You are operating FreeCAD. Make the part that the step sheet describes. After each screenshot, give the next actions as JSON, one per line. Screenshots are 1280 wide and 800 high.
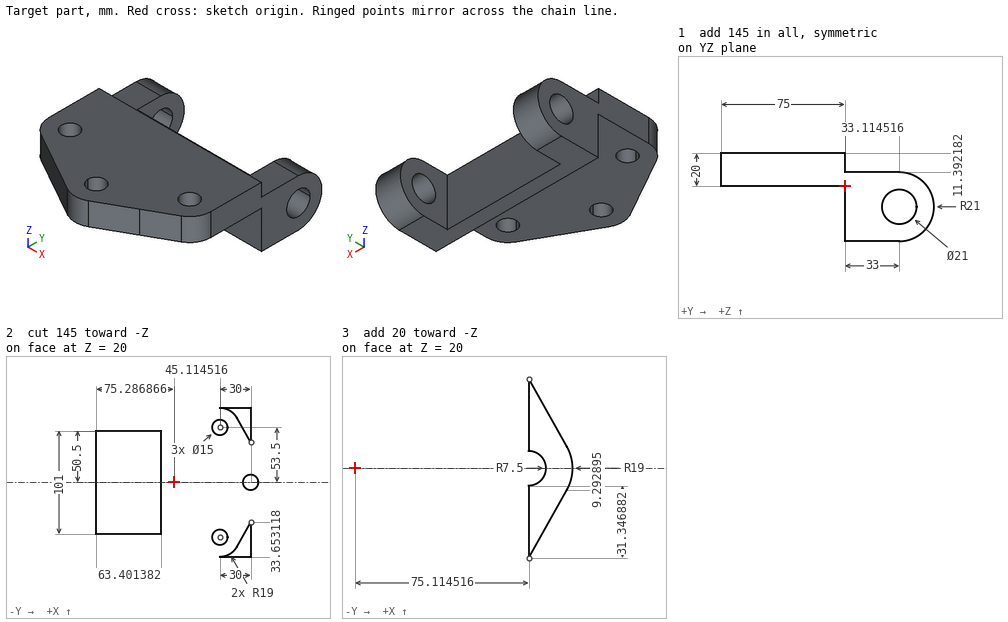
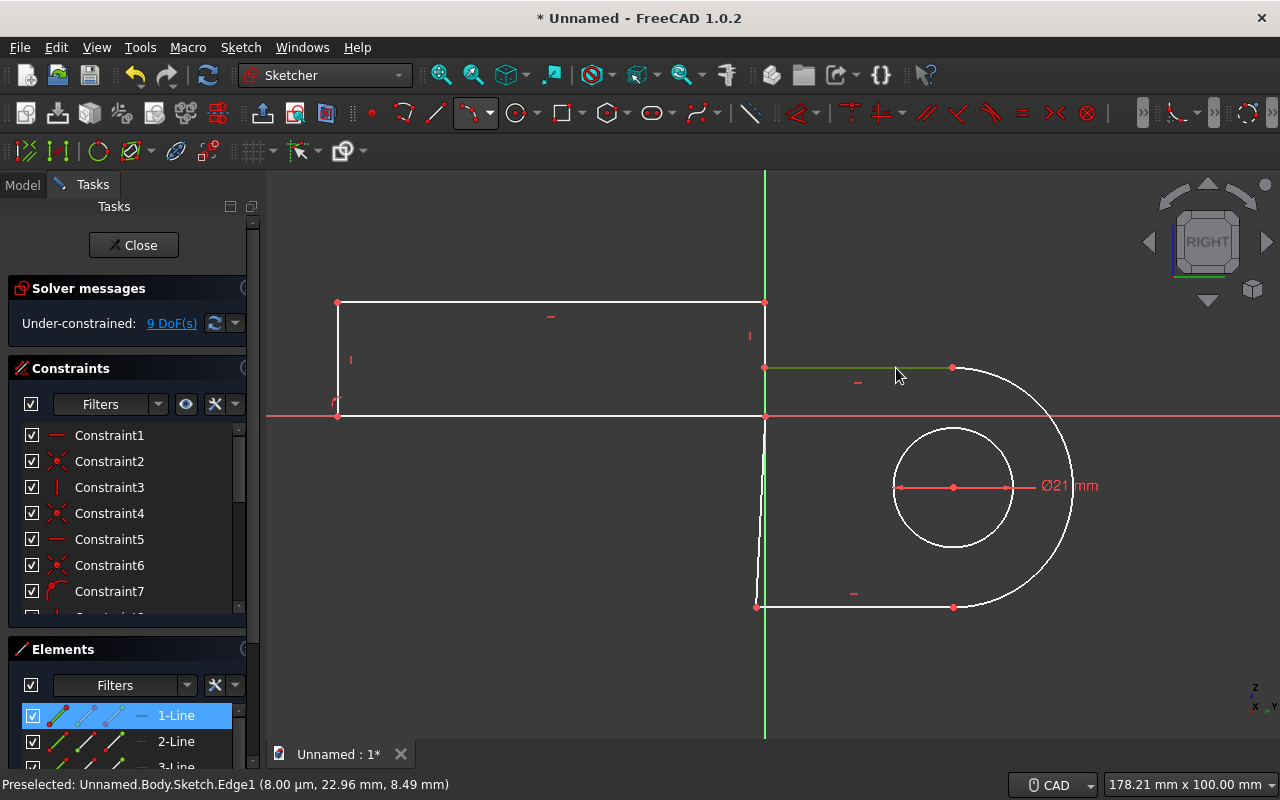
{"action": "left_click", "coordinate": [1050, 558]}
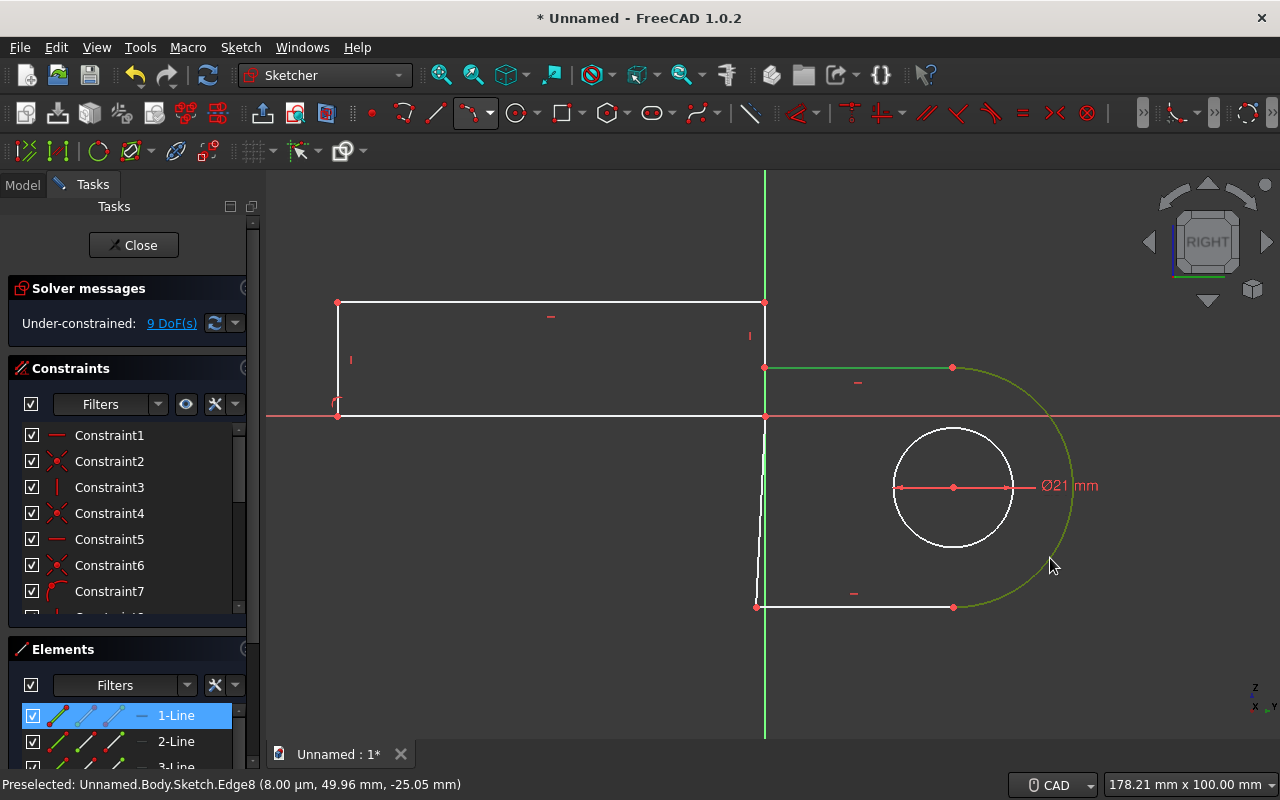
{"action": "left_click", "coordinate": [992, 114]}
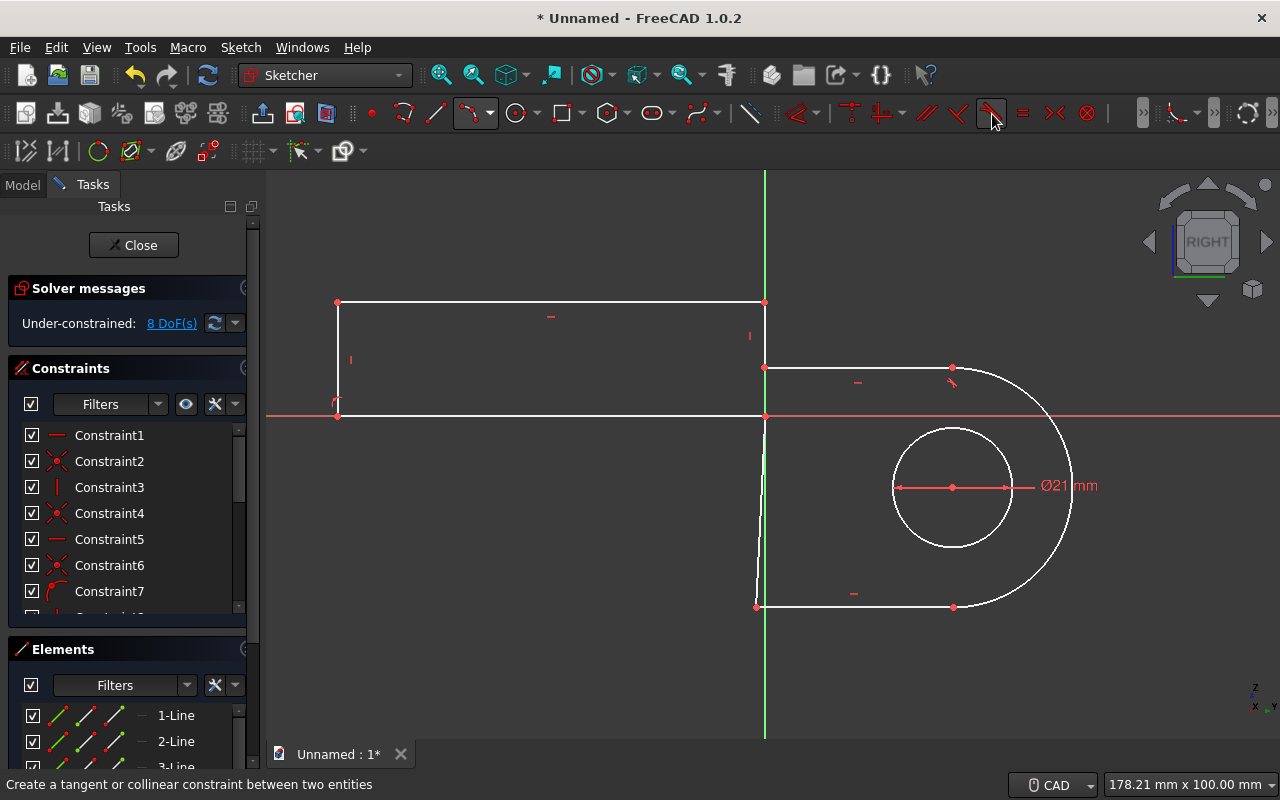
{"action": "left_click", "coordinate": [815, 607]}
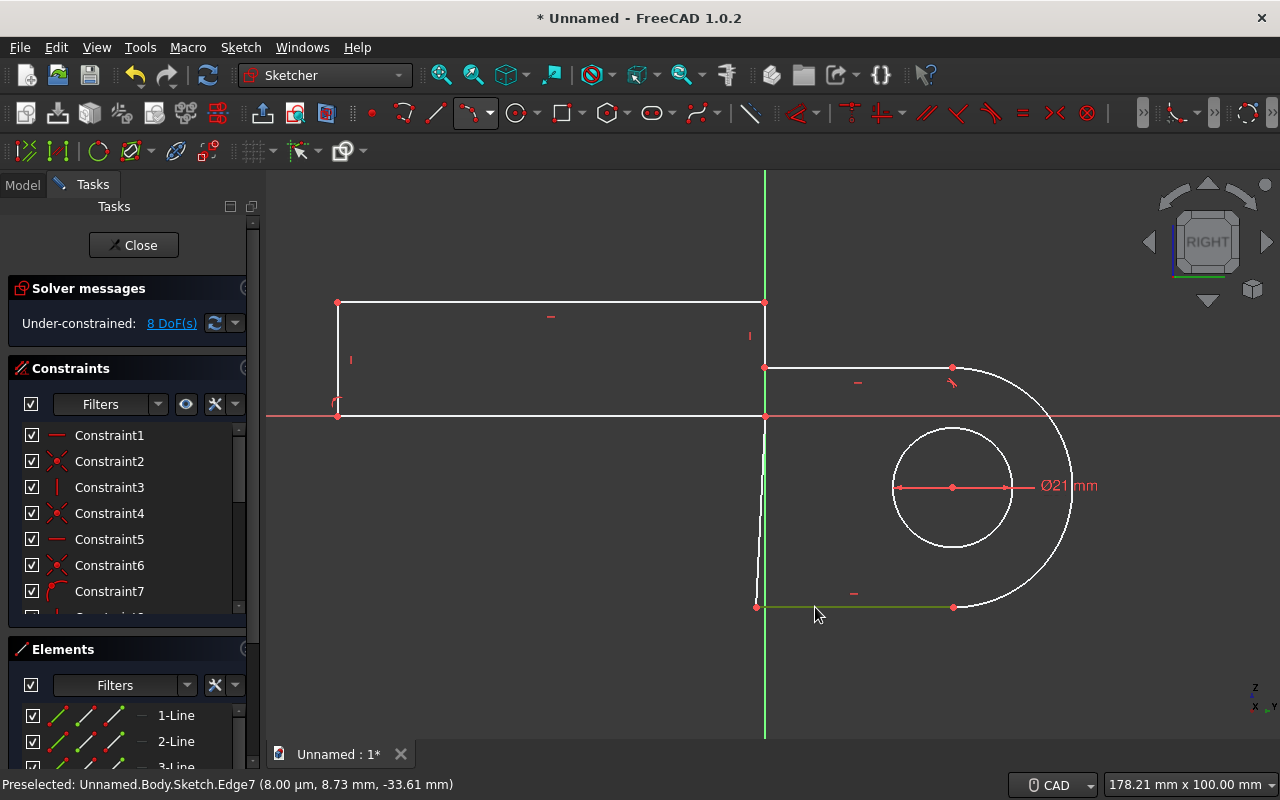
{"action": "left_click", "coordinate": [1050, 558]}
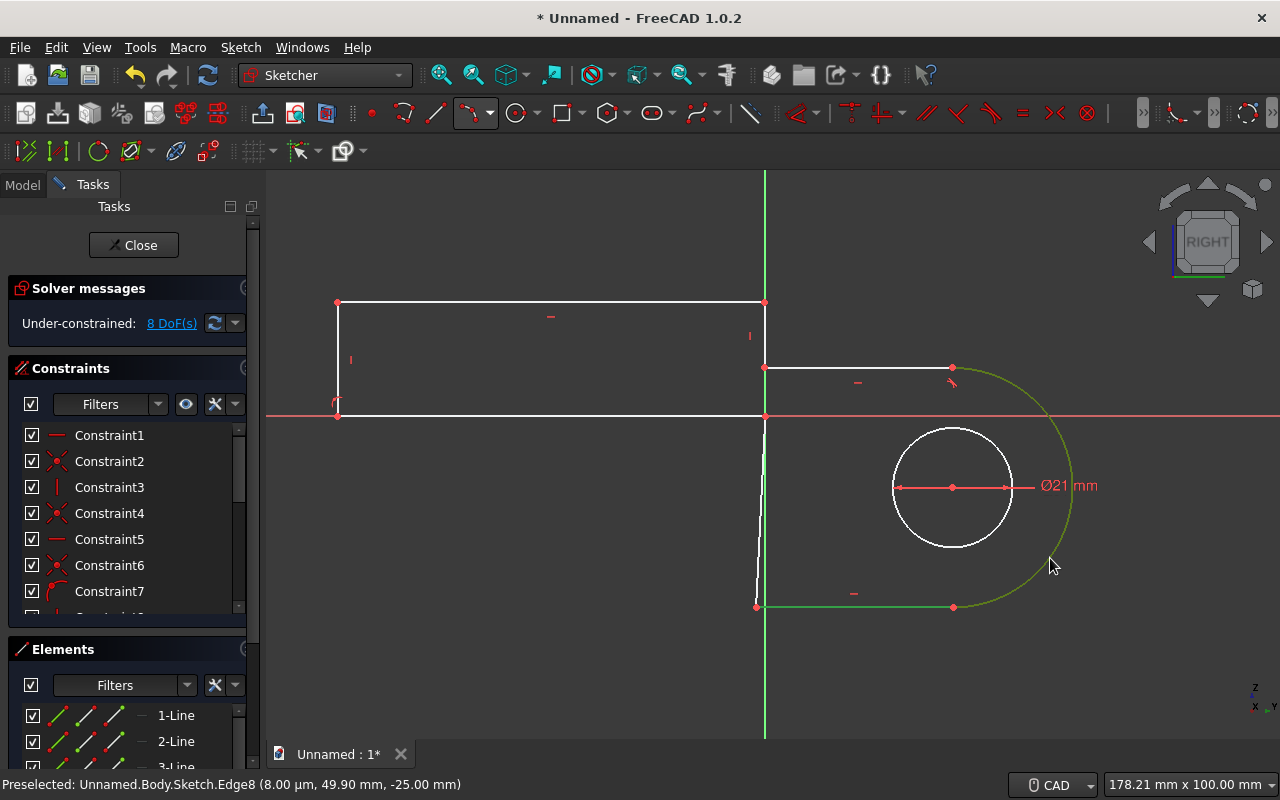
{"action": "left_click", "coordinate": [992, 114]}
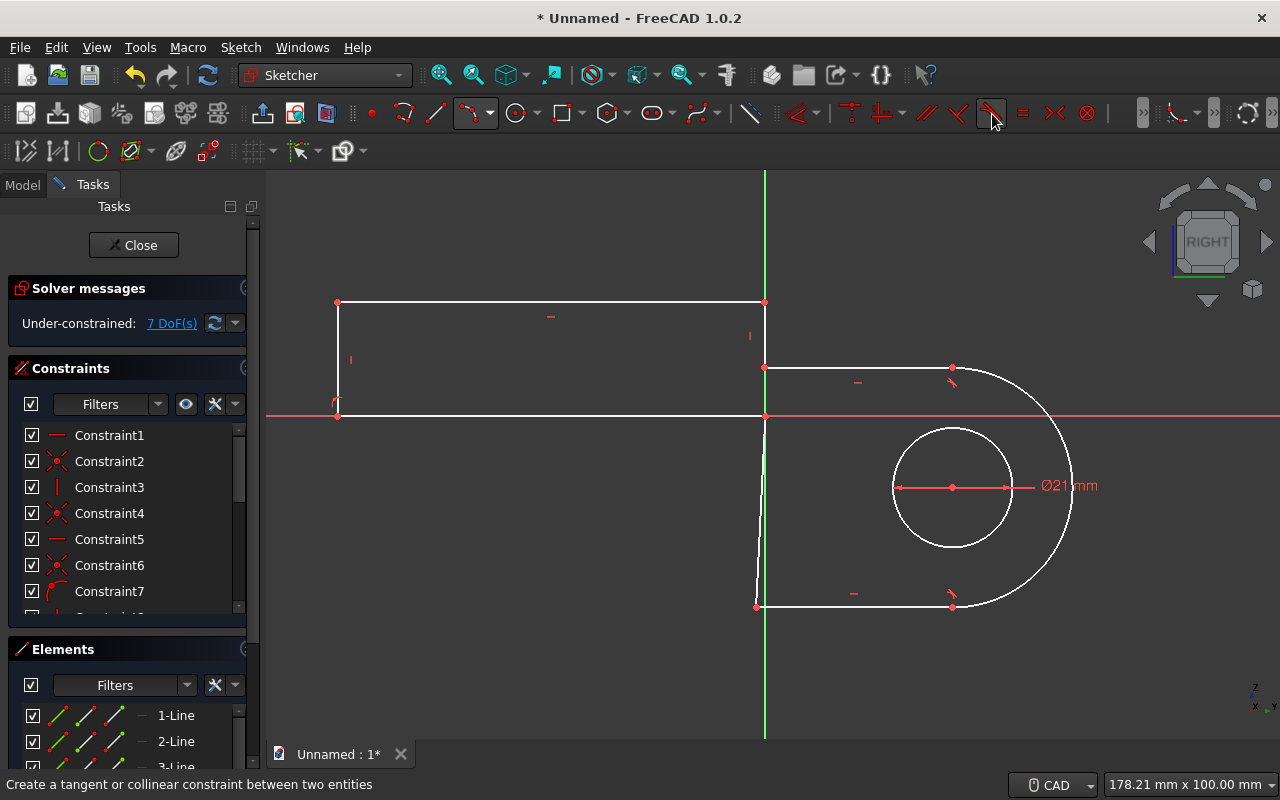
{"action": "left_click", "coordinate": [763, 474]}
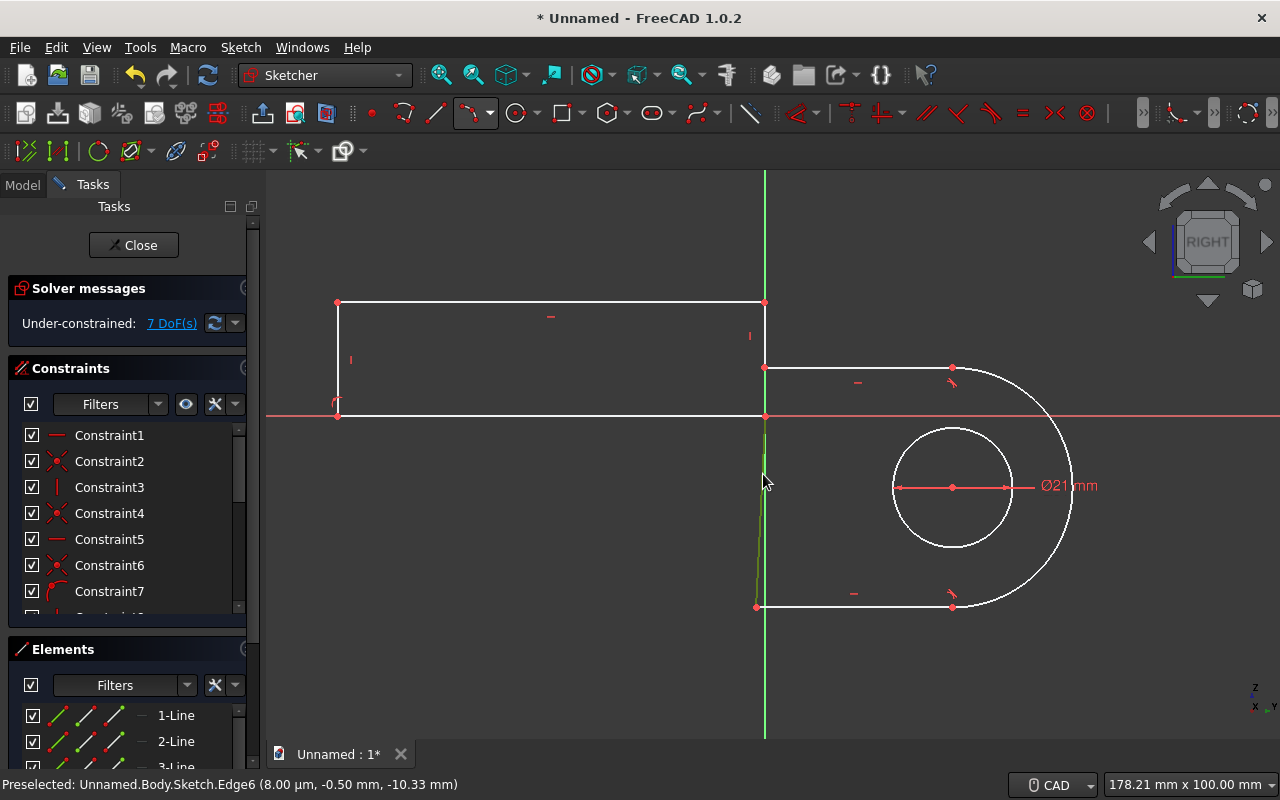
{"action": "key", "text": "v"}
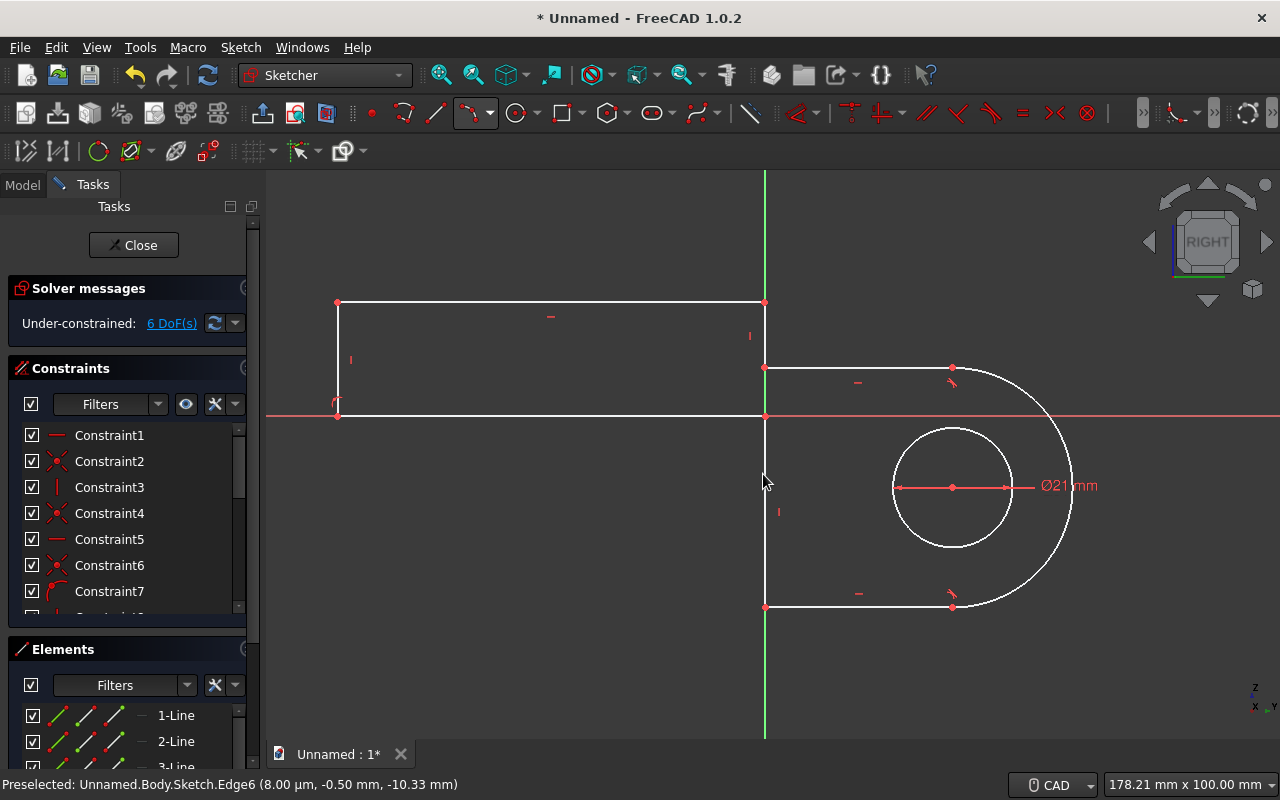
{"action": "left_click", "coordinate": [796, 114]}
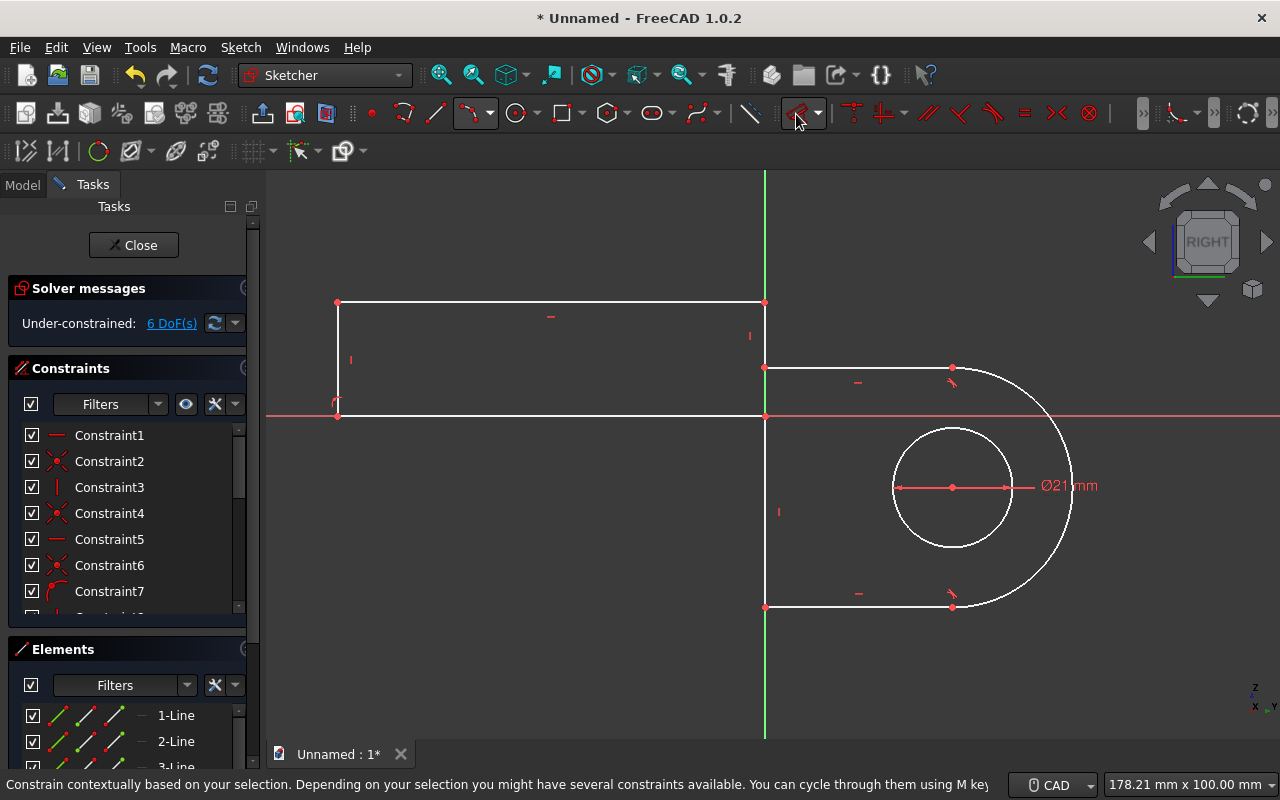
{"action": "left_click", "coordinate": [1050, 558]}
{"action": "left_click", "coordinate": [1076, 577]}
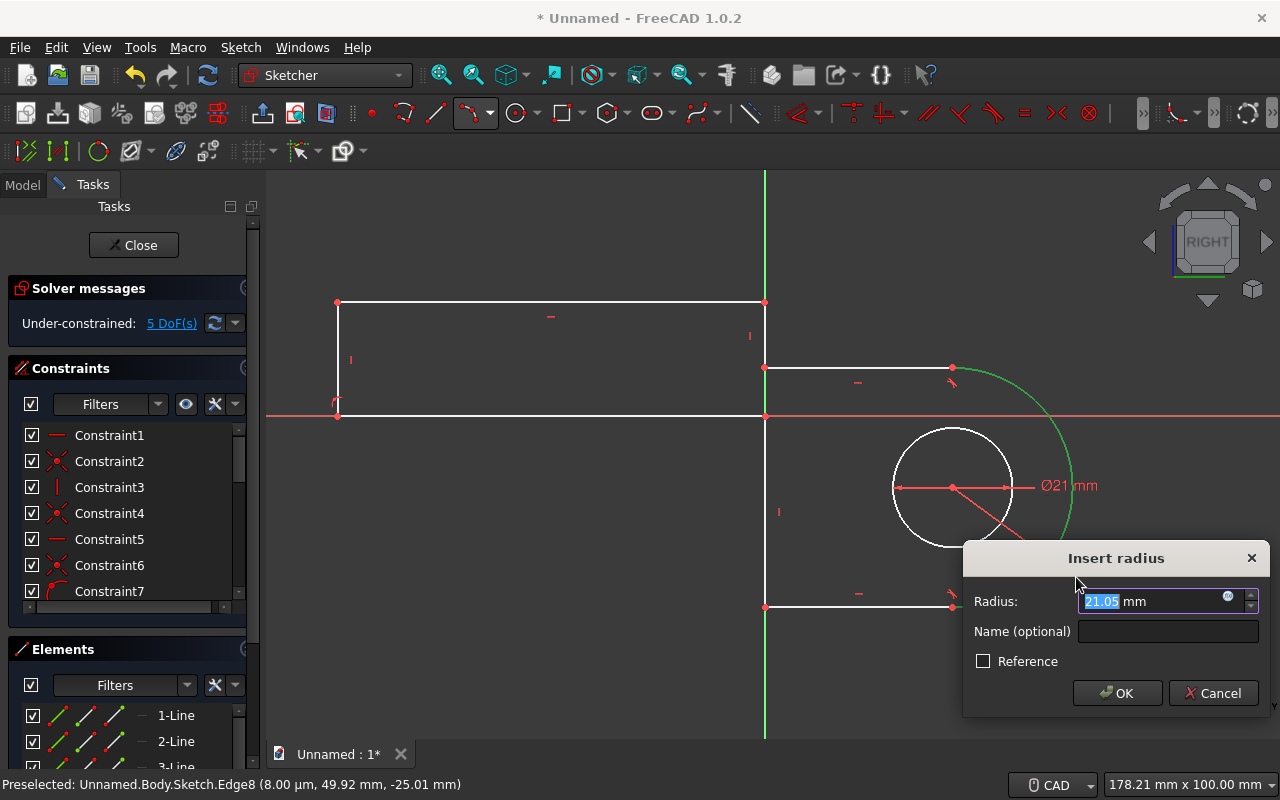
{"action": "type", "text": "21"}
{"action": "key", "text": "Return"}